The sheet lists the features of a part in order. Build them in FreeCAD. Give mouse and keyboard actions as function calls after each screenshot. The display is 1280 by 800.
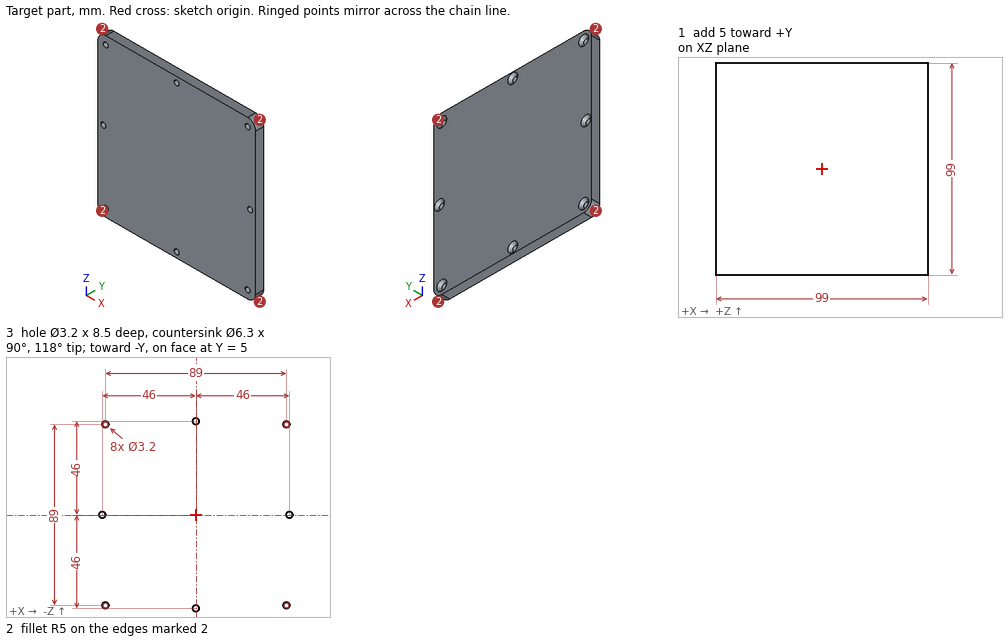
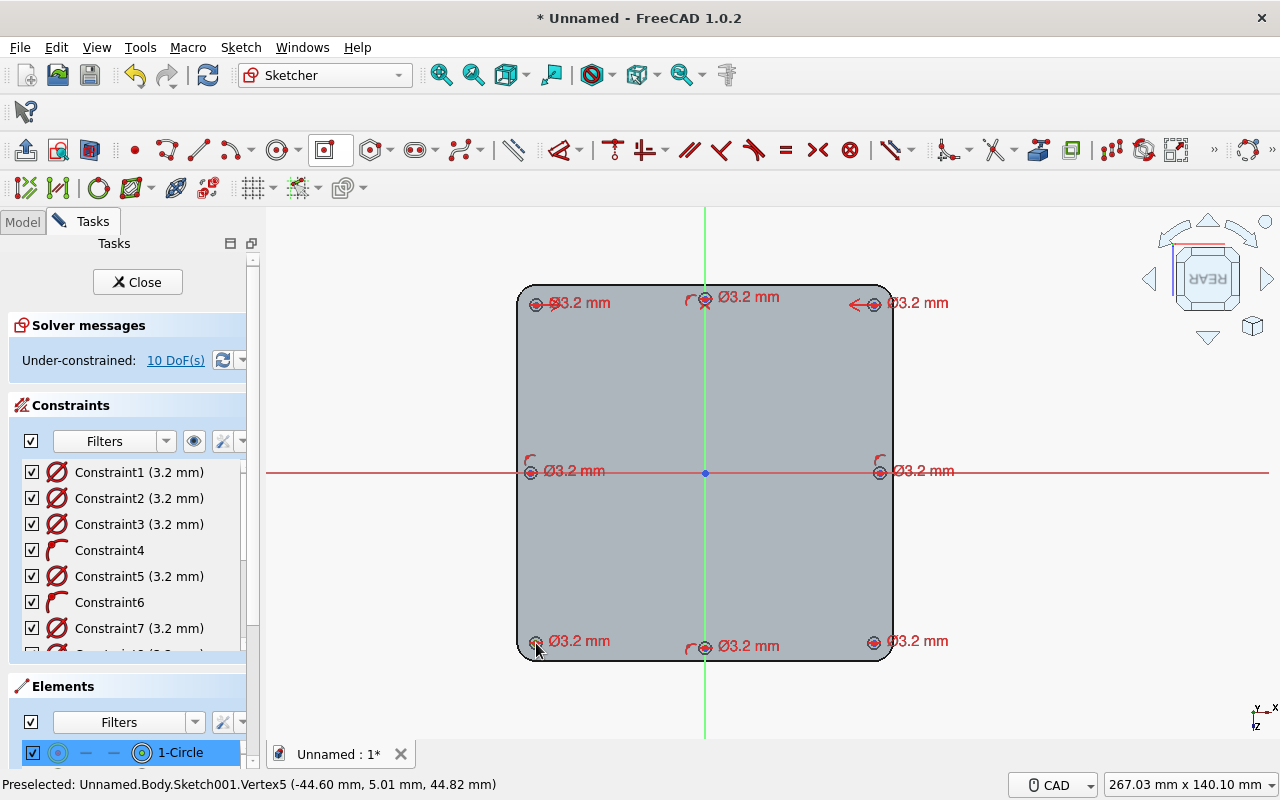
click(353, 473)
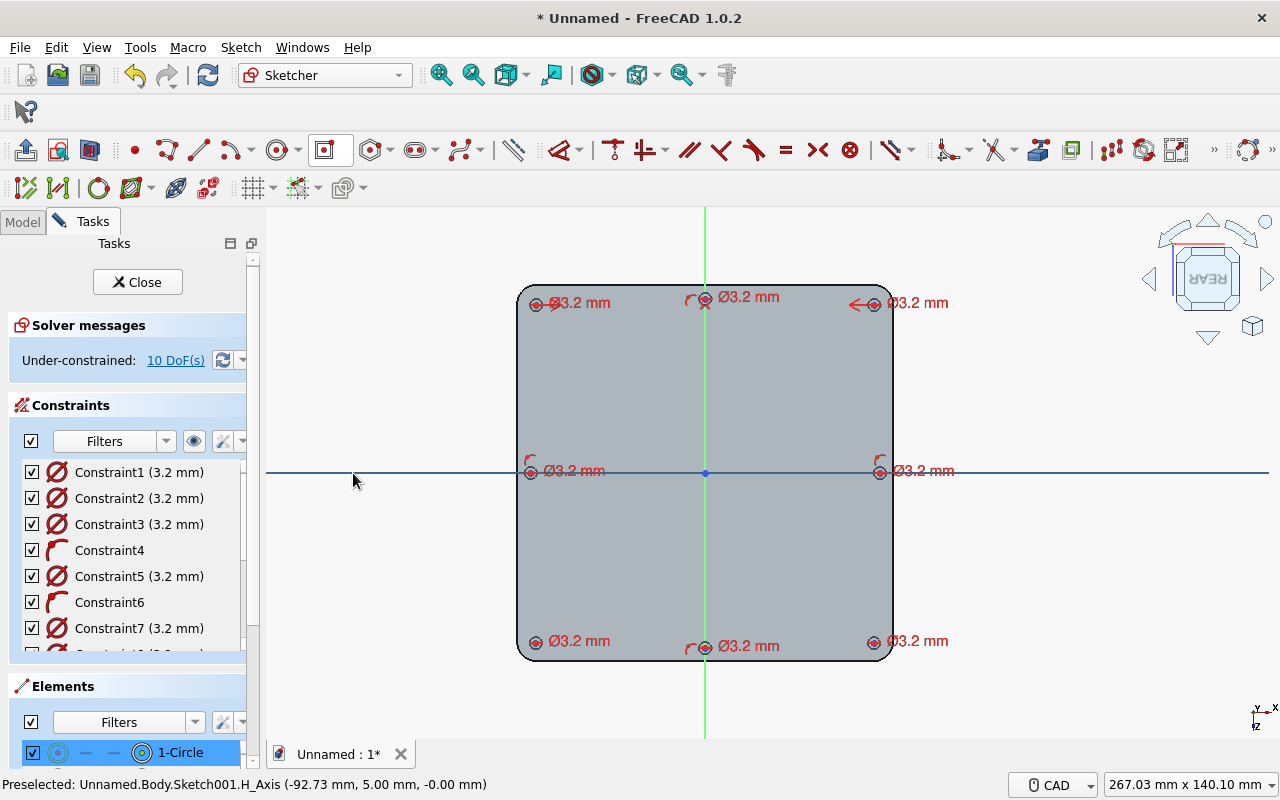
key(s)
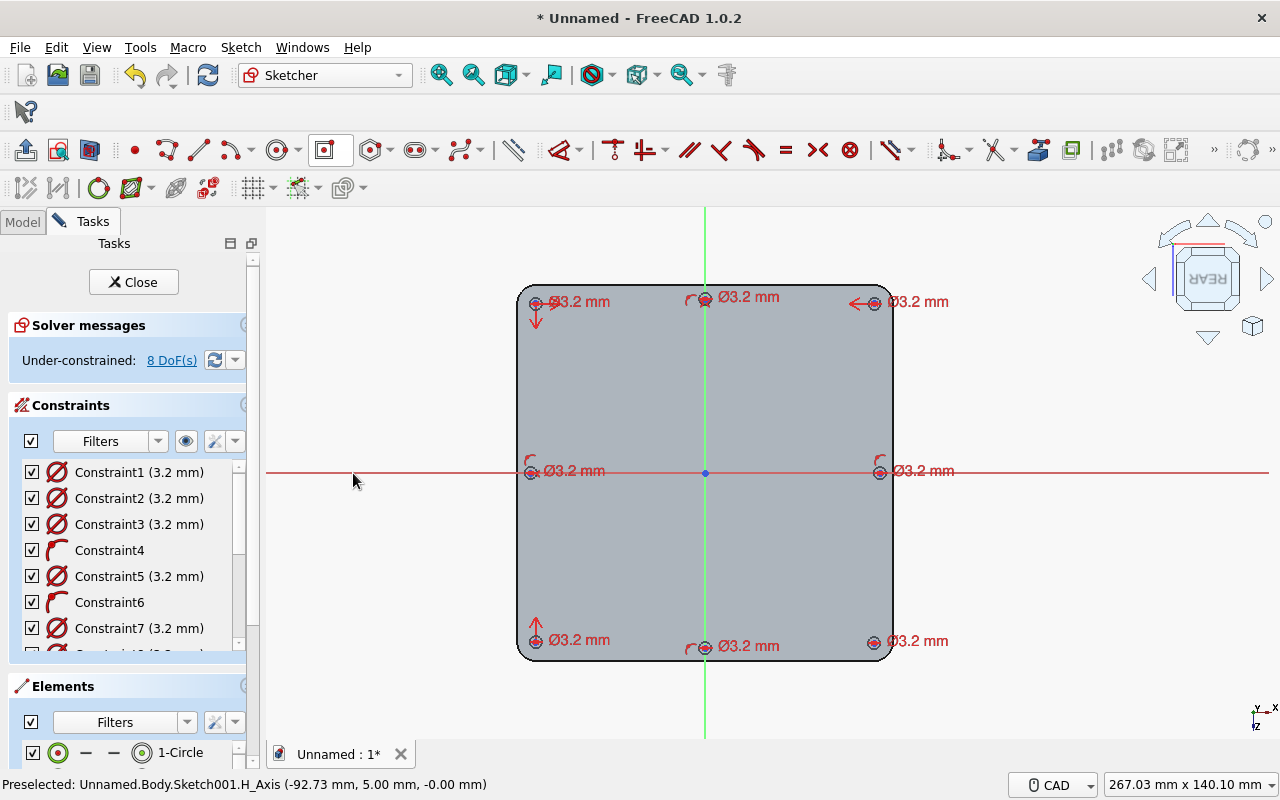
click(874, 304)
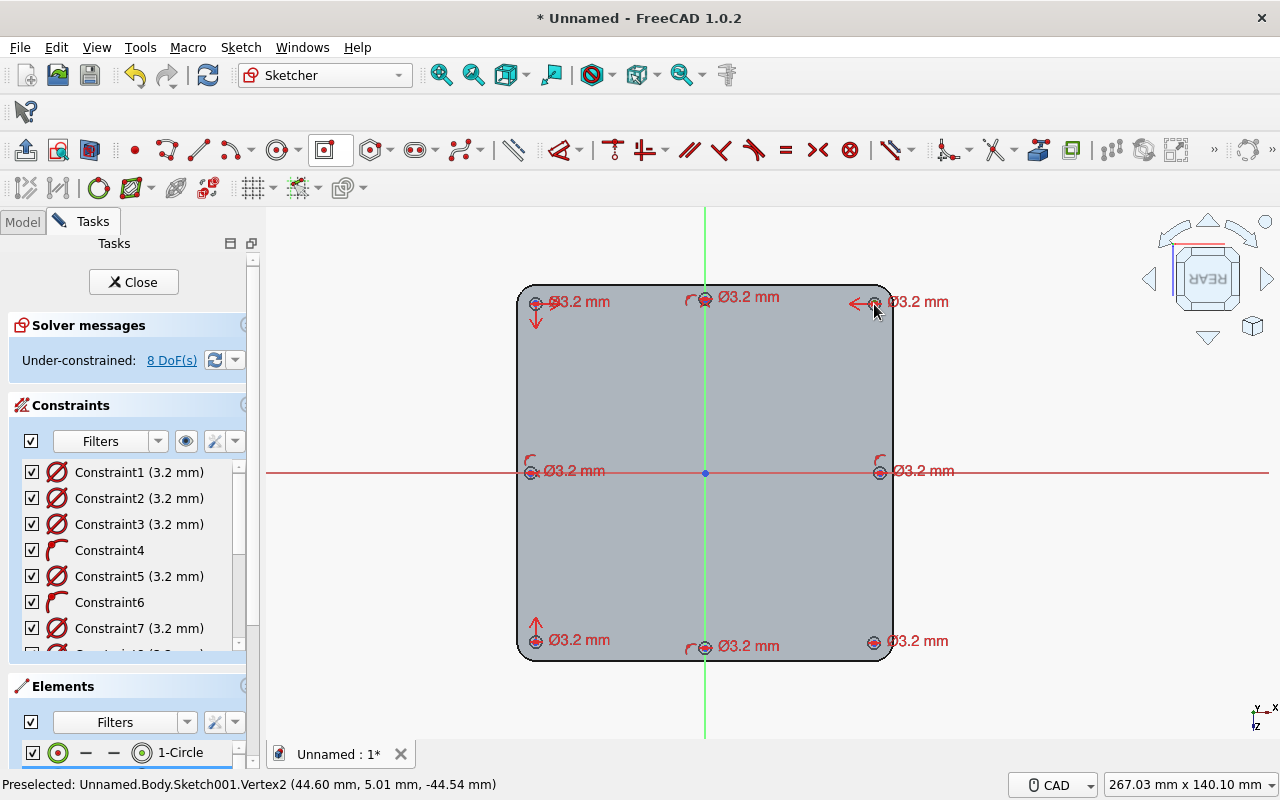
click(874, 643)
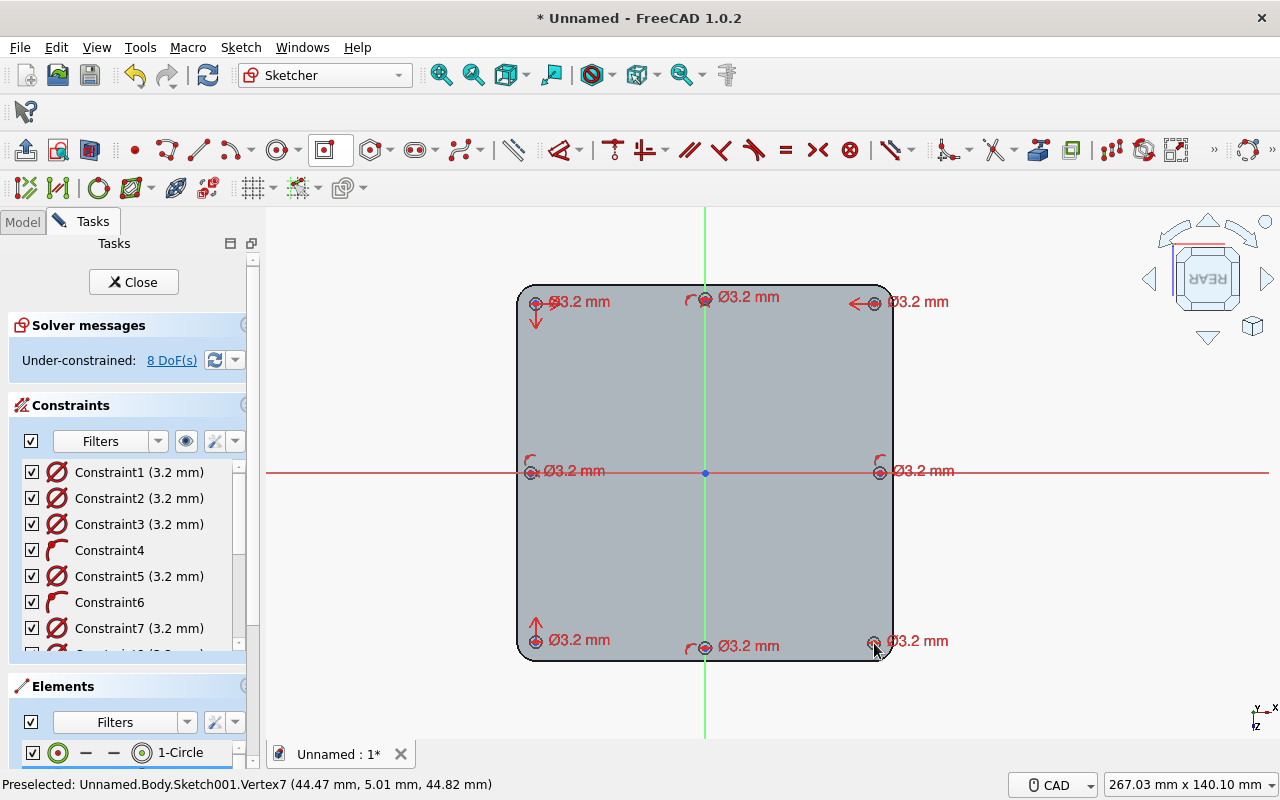
click(353, 473)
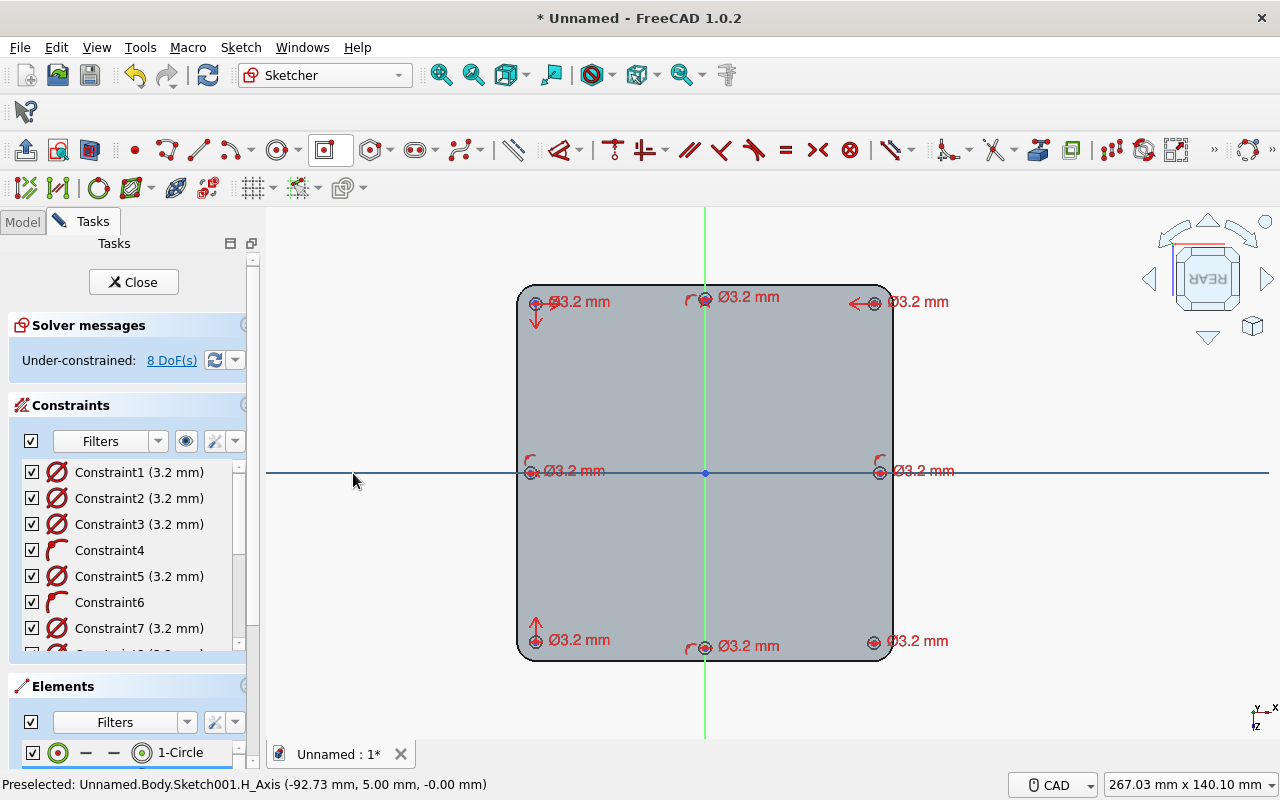
key(s)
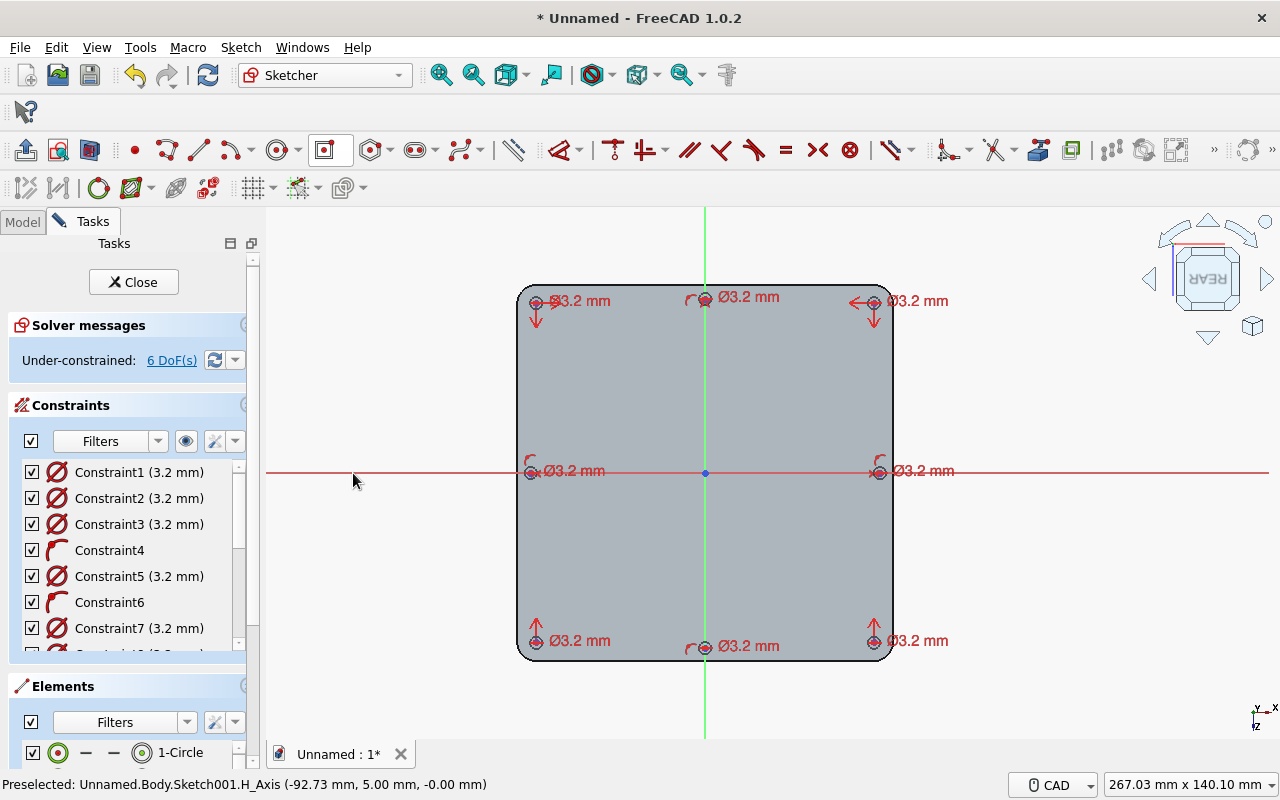
click(560, 150)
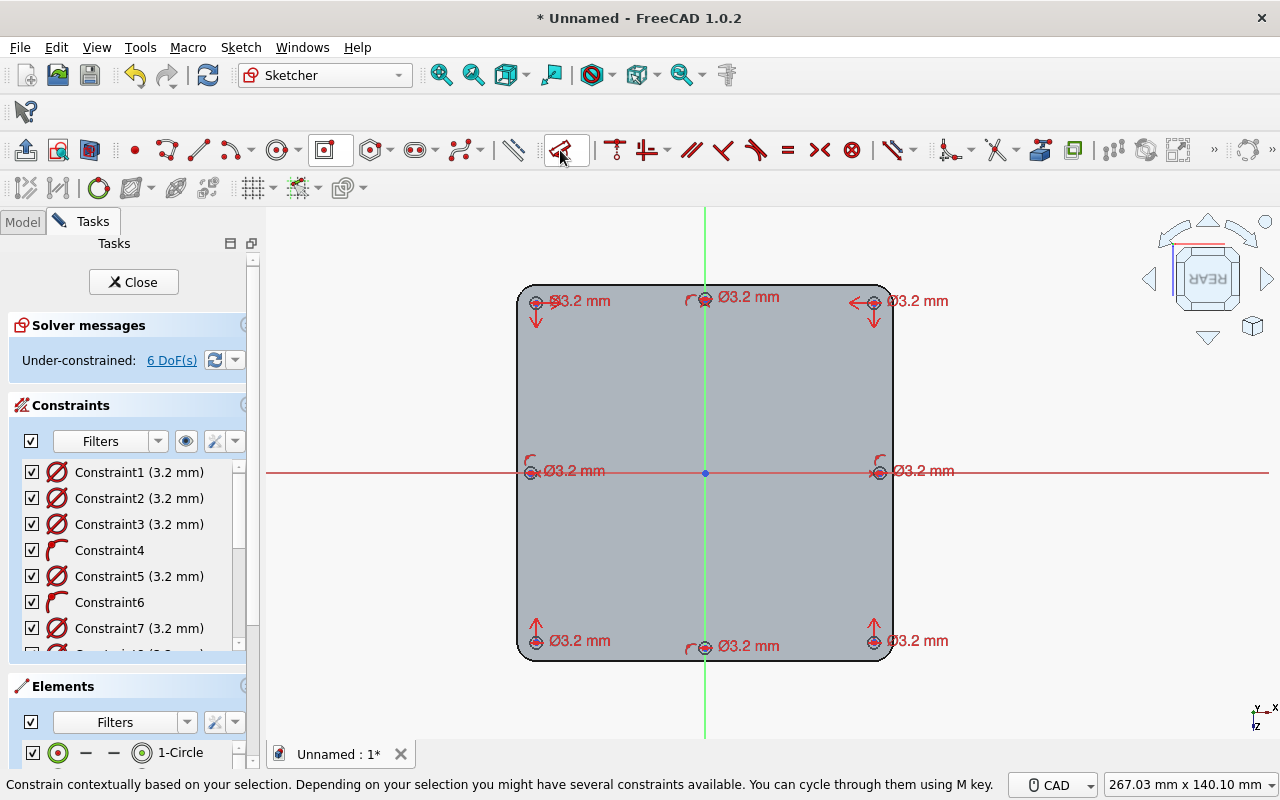
click(705, 299)
click(739, 386)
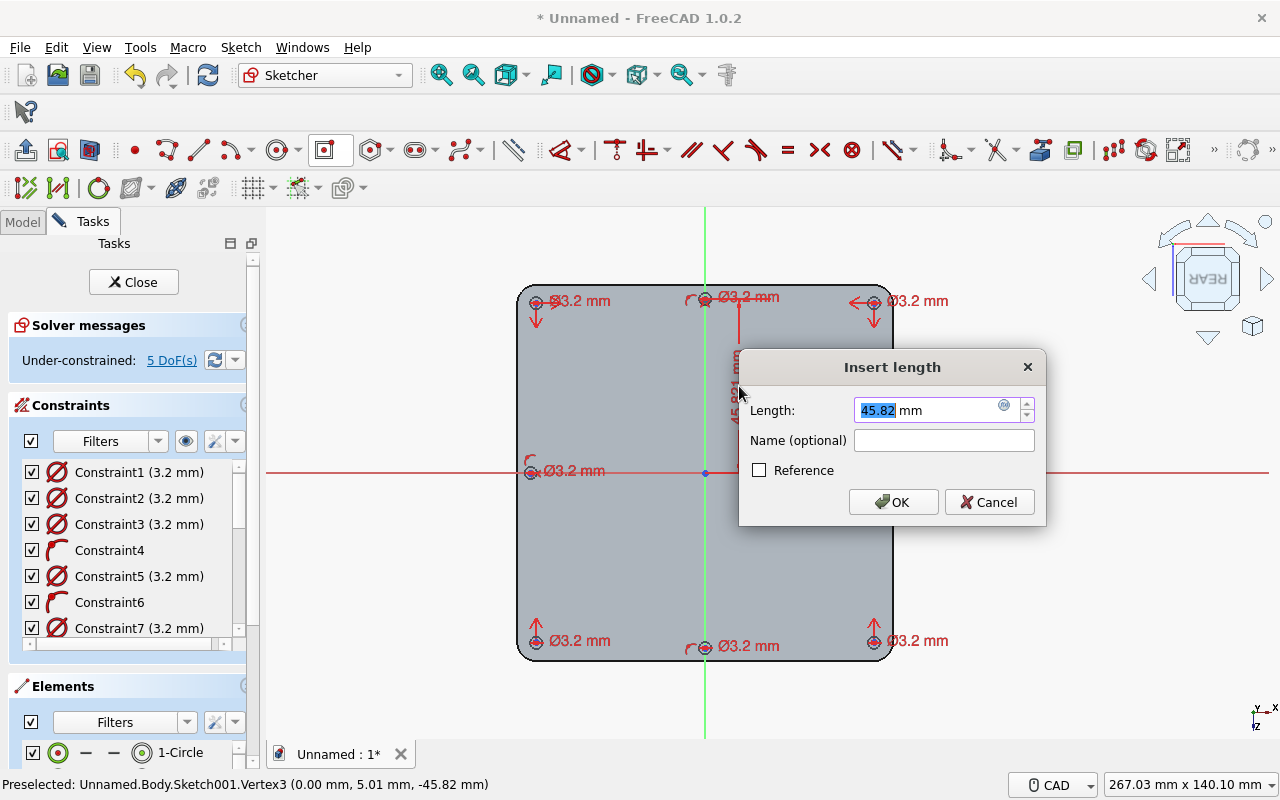
text(46)
key(Return)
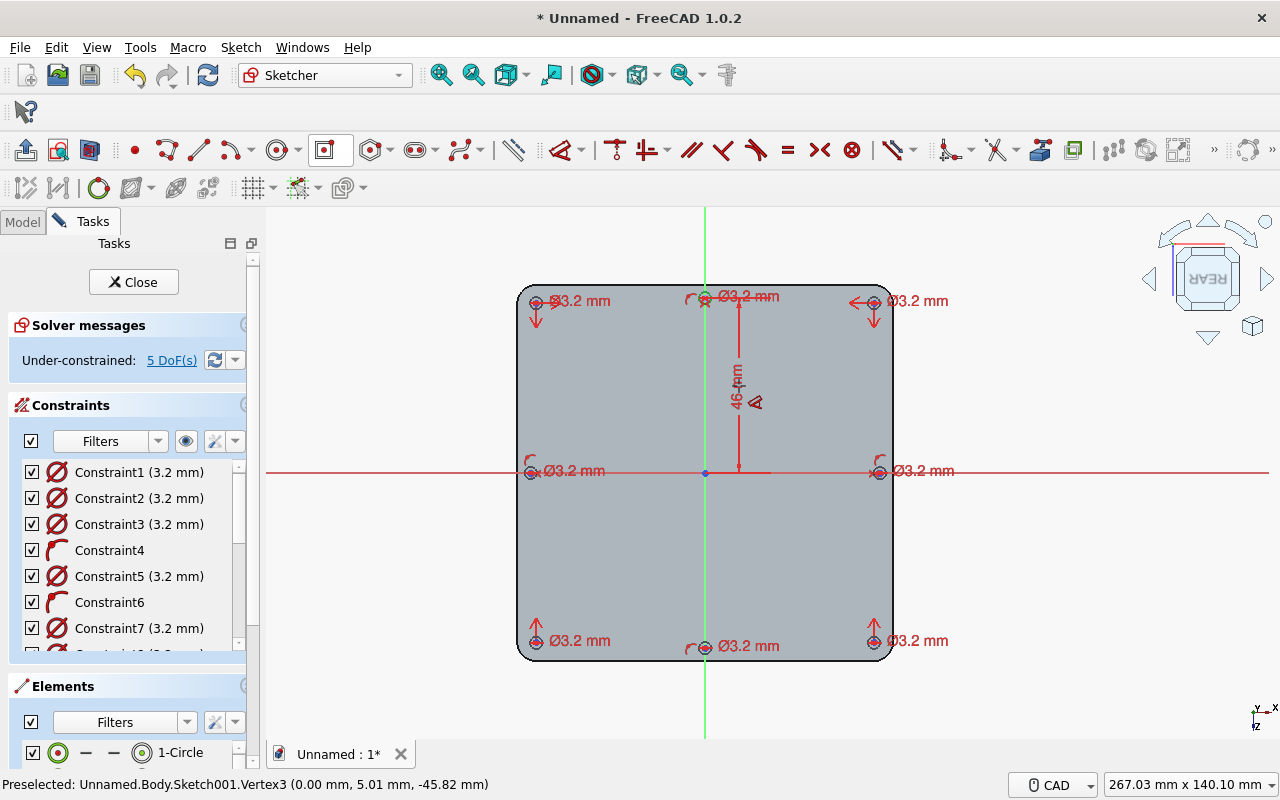
click(531, 473)
click(618, 507)